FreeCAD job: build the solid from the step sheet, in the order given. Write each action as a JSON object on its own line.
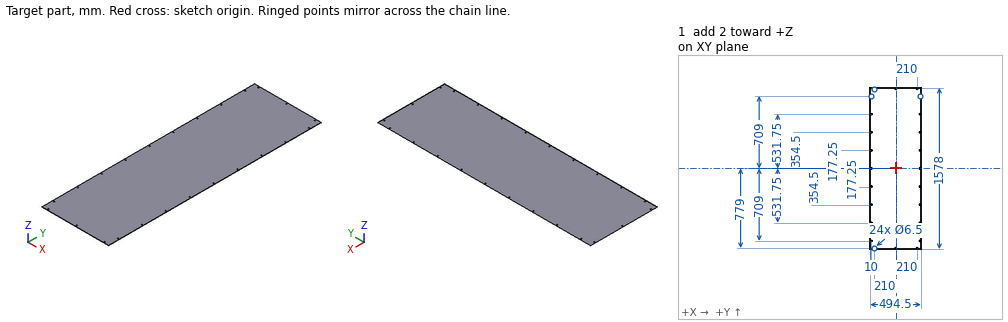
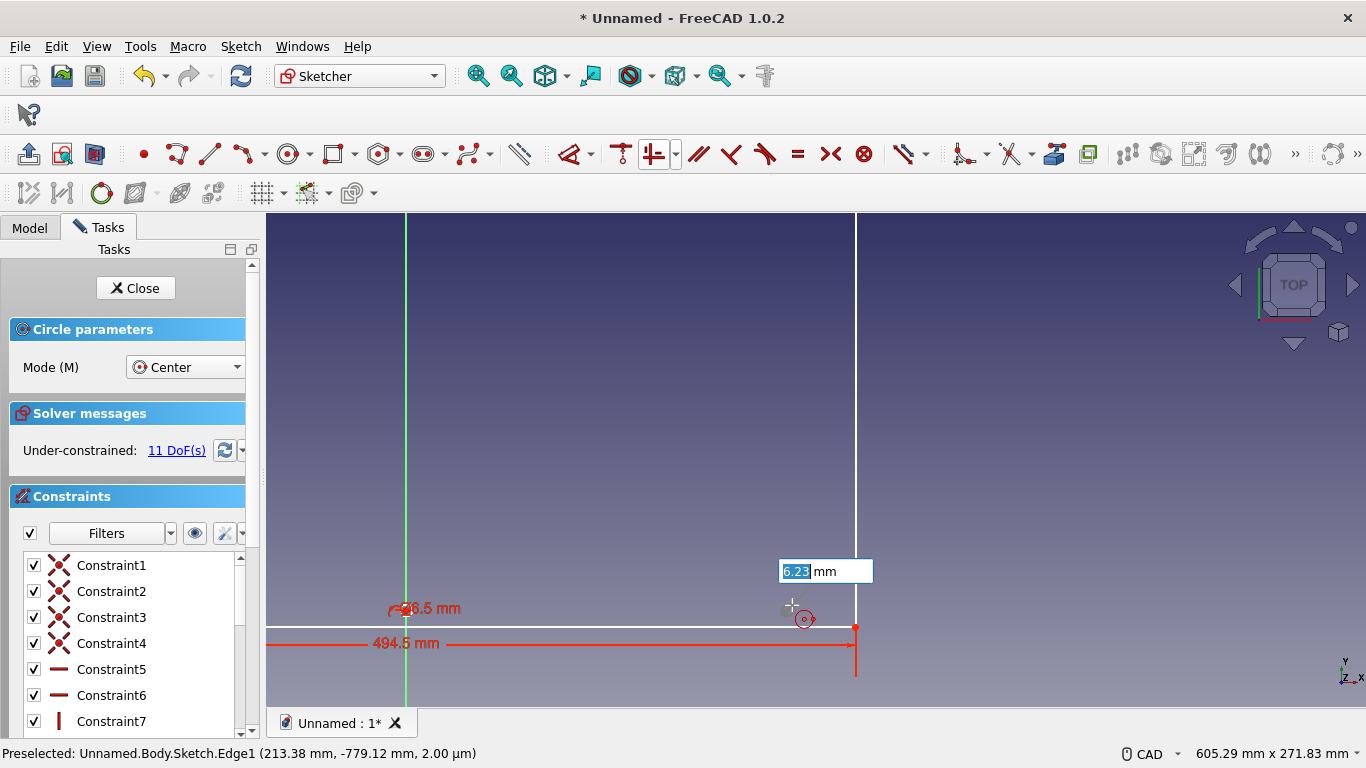
{"action": "type", "text": "6.5"}
{"action": "key", "text": "Return"}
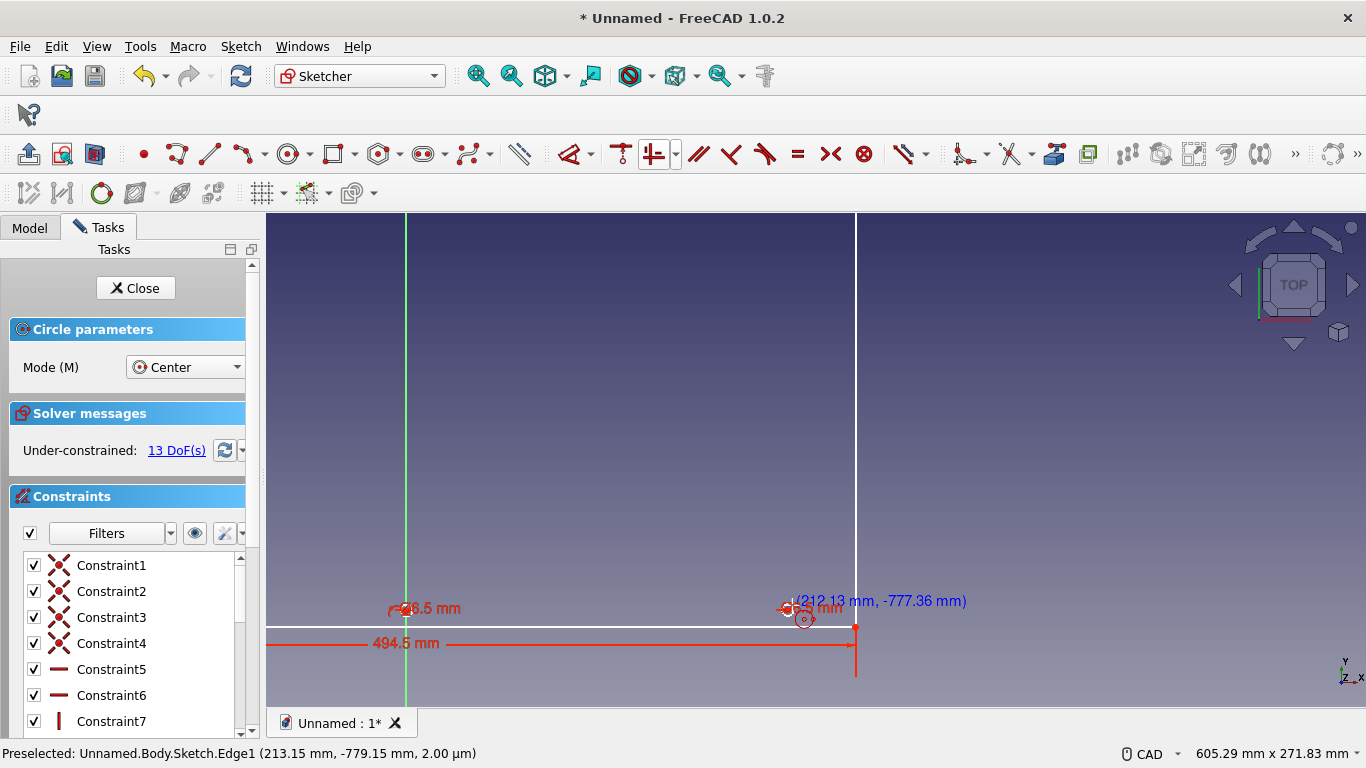
{"action": "scroll", "coordinate": [838, 482], "scroll_direction": "up", "scroll_amount": 7}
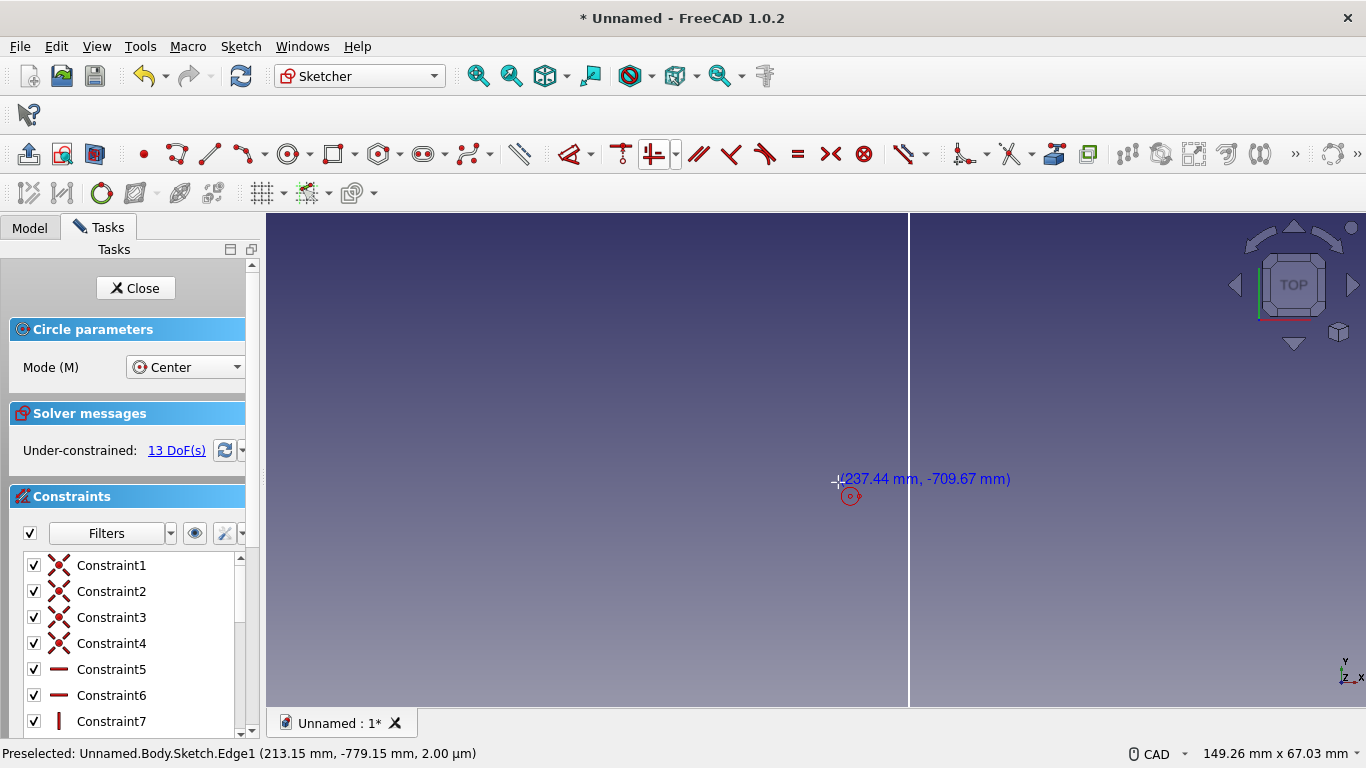
{"action": "scroll", "coordinate": [794, 606], "scroll_direction": "down", "scroll_amount": 18}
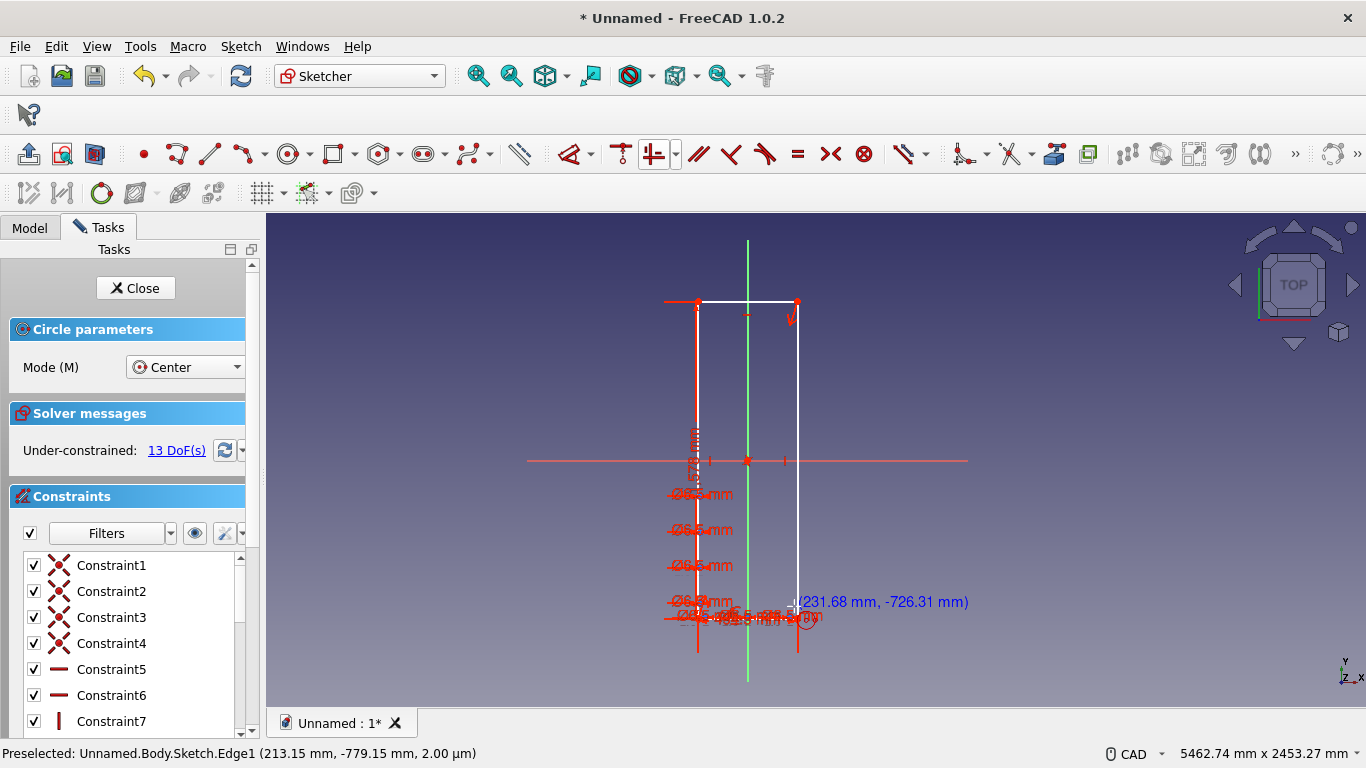
{"action": "scroll", "coordinate": [796, 603], "scroll_direction": "up", "scroll_amount": 11}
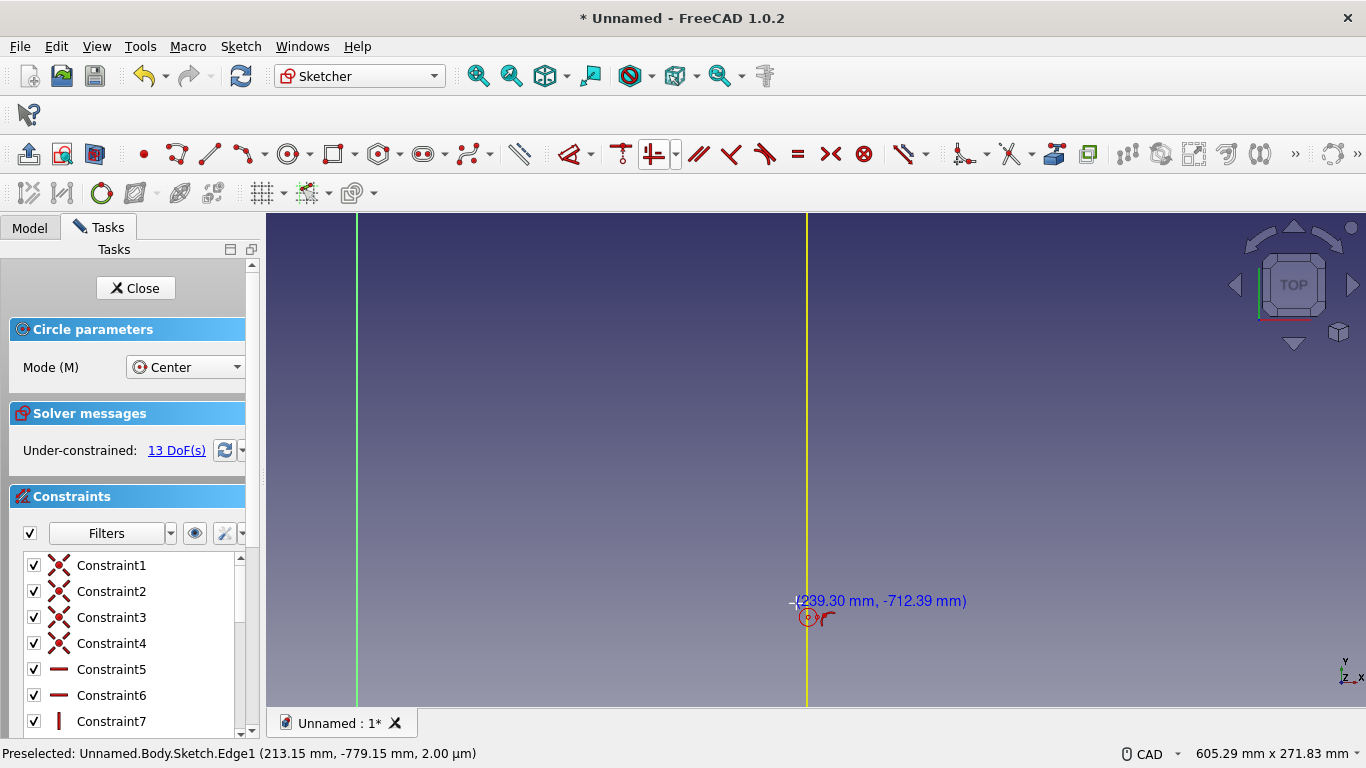
{"action": "left_click", "coordinate": [788, 600]}
{"action": "mouse_move", "coordinate": [784, 595]}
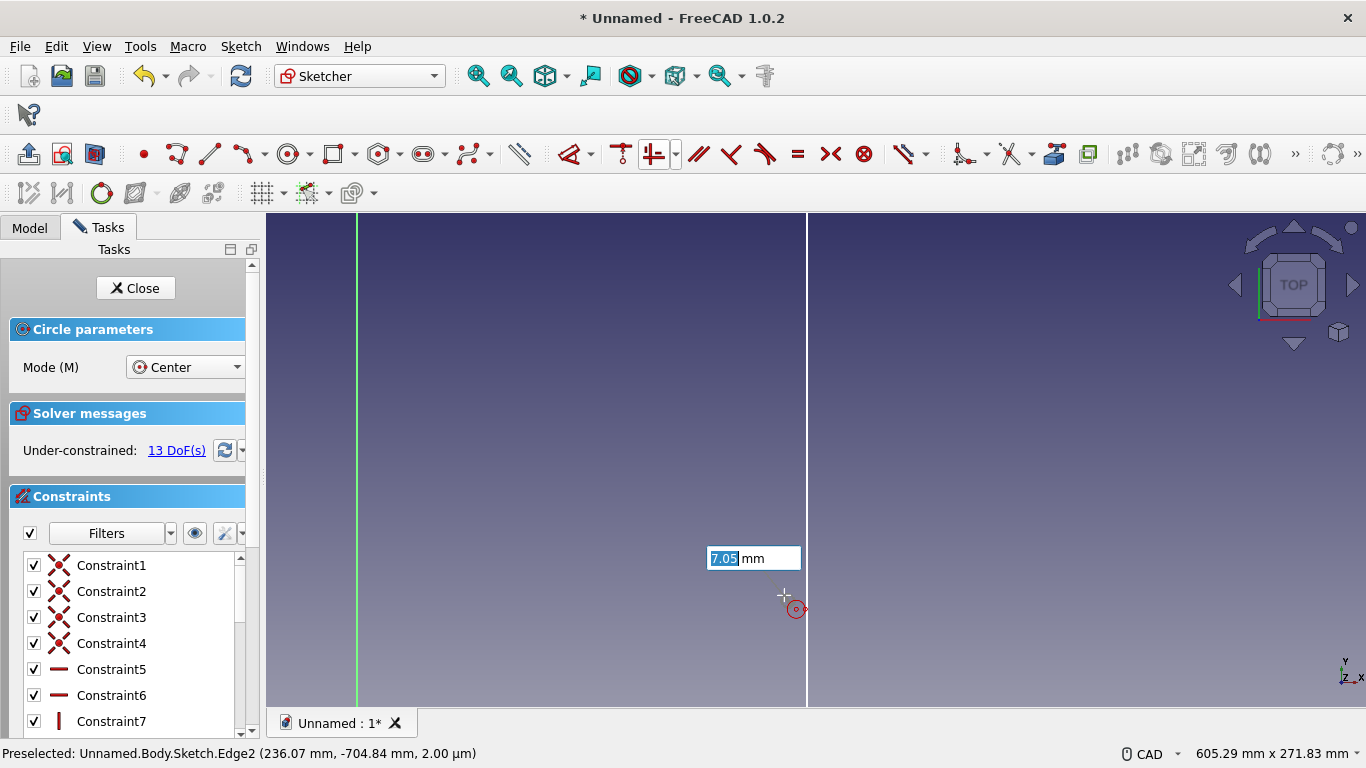
{"action": "type", "text": "6.5"}
{"action": "key", "text": "Return"}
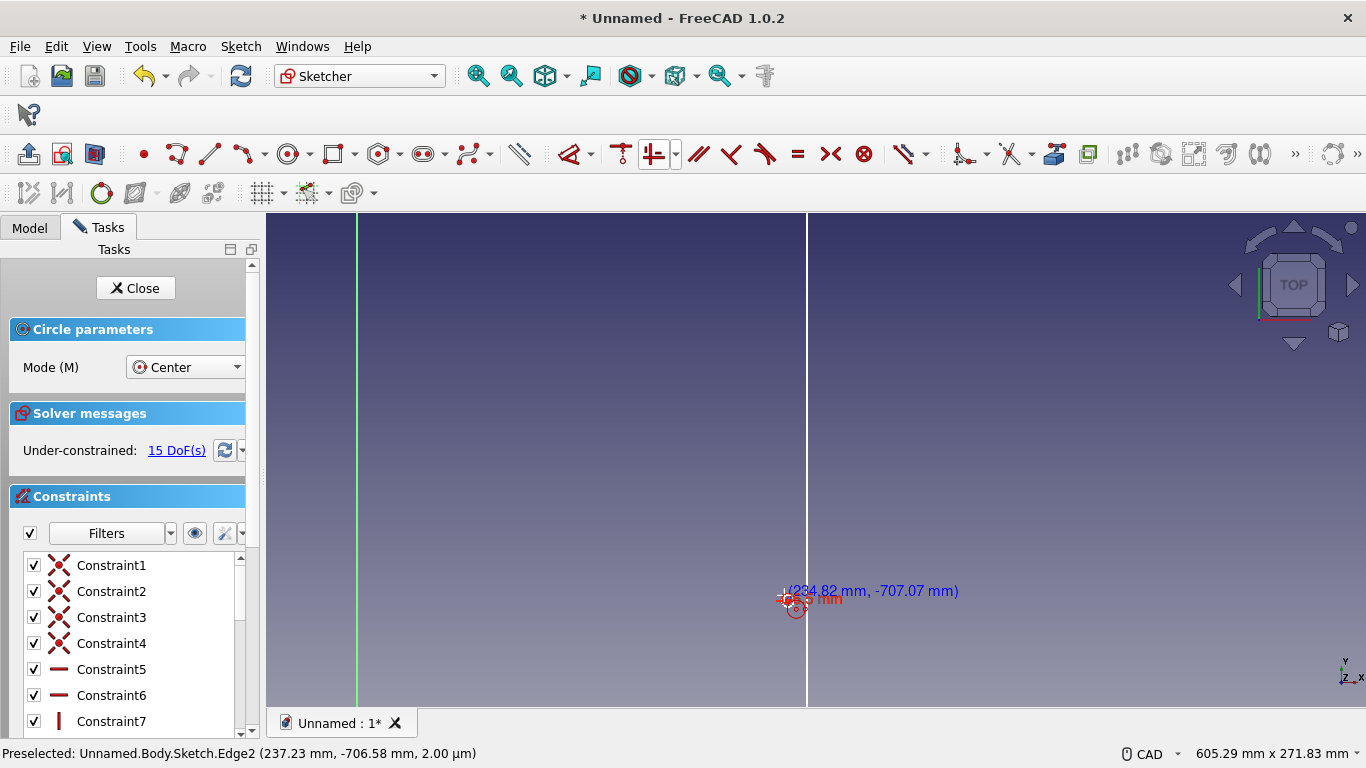
{"action": "scroll", "coordinate": [788, 277], "scroll_direction": "up", "scroll_amount": 7}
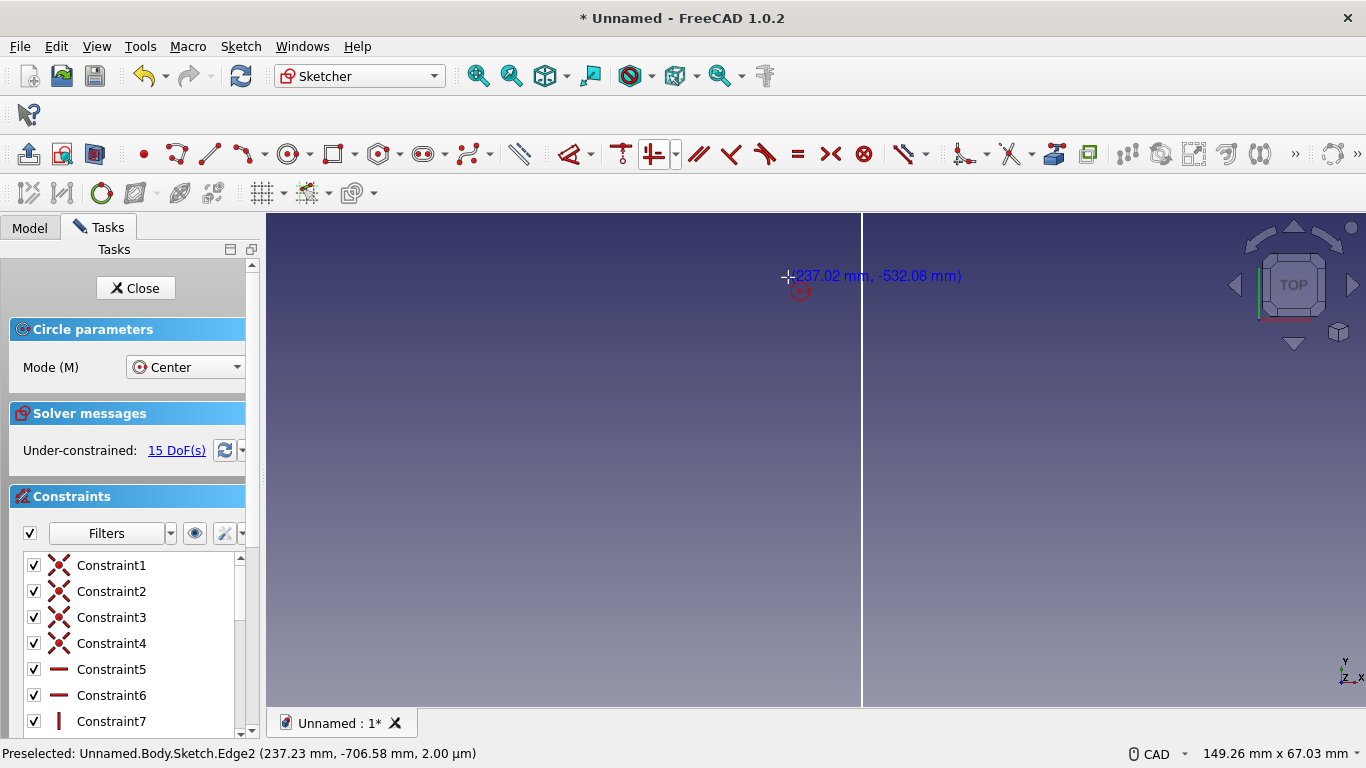
{"action": "scroll", "coordinate": [795, 575], "scroll_direction": "down", "scroll_amount": 18}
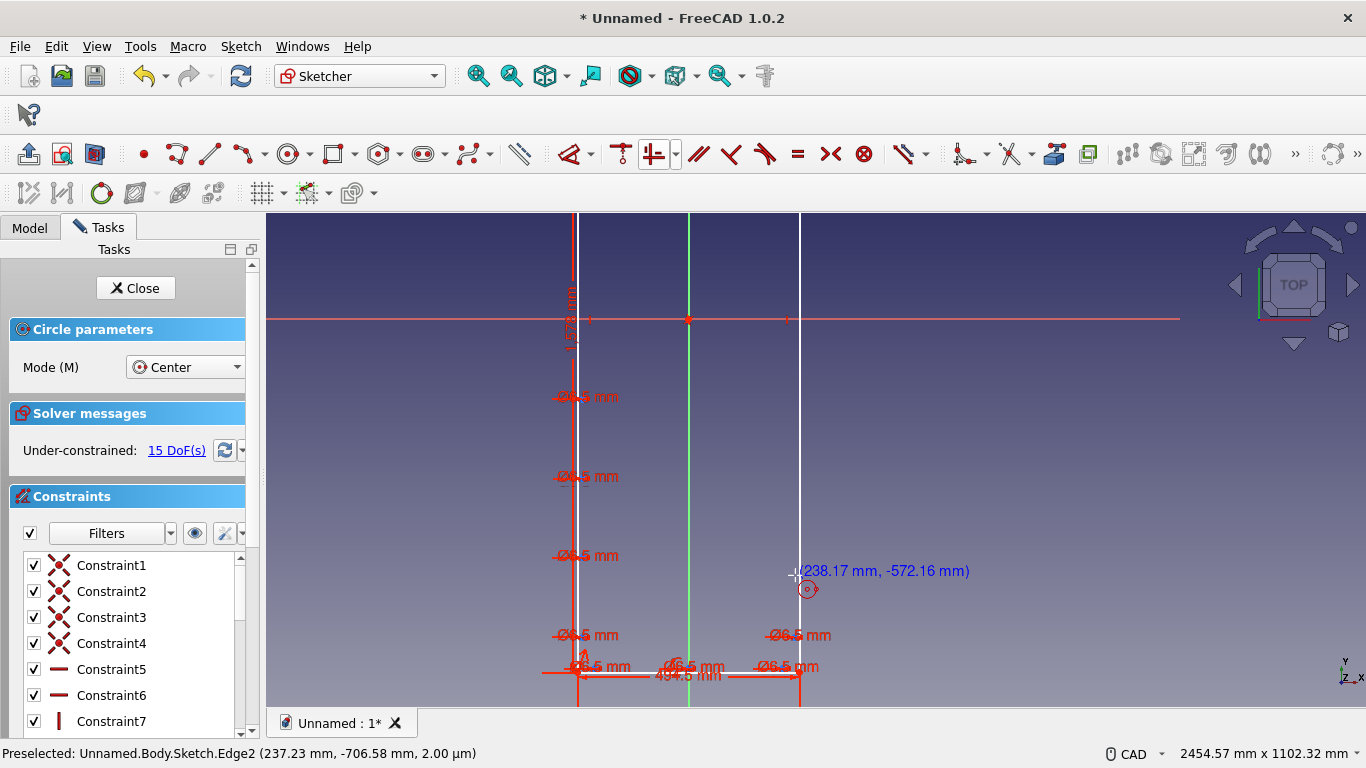
{"action": "scroll", "coordinate": [795, 568], "scroll_direction": "up", "scroll_amount": 11}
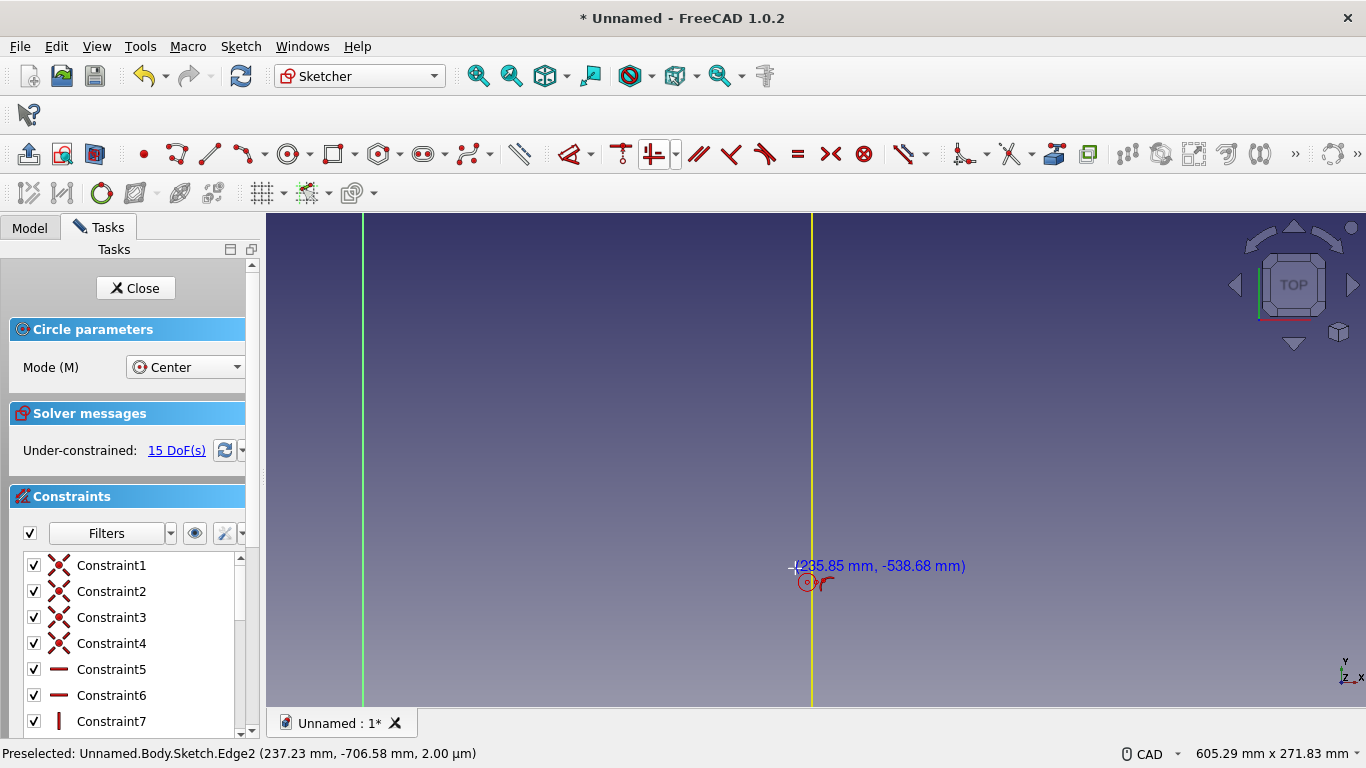
{"action": "left_click", "coordinate": [794, 559]}
{"action": "mouse_move", "coordinate": [790, 554]}